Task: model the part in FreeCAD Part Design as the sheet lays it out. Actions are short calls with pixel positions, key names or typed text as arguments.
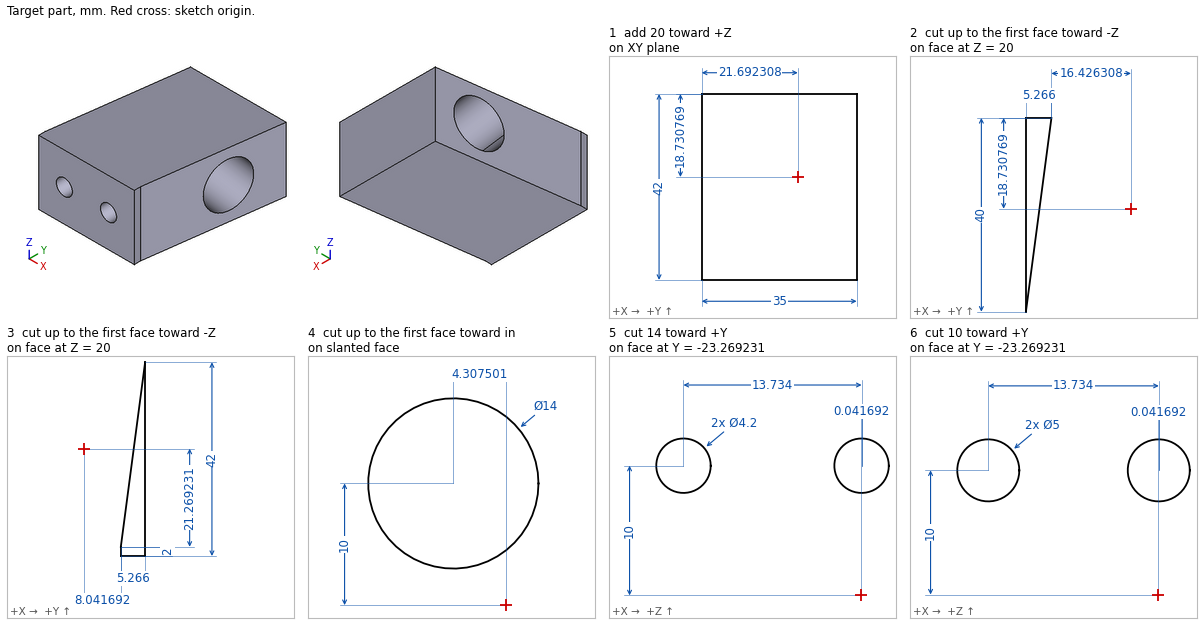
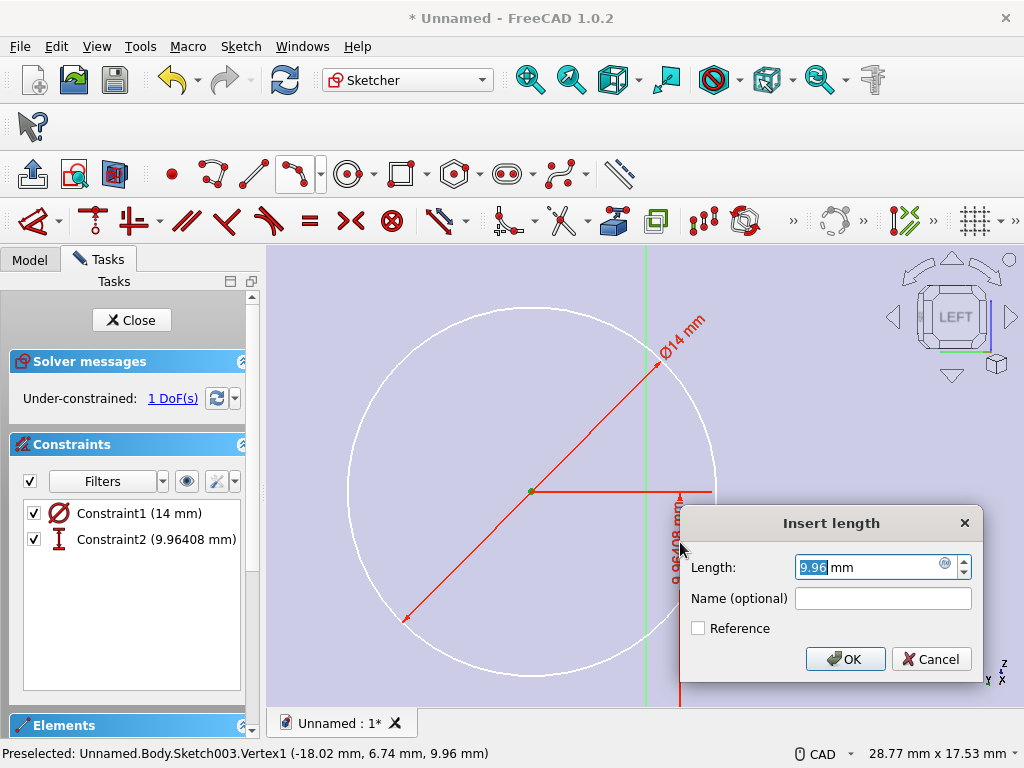
text(10)
key(Return)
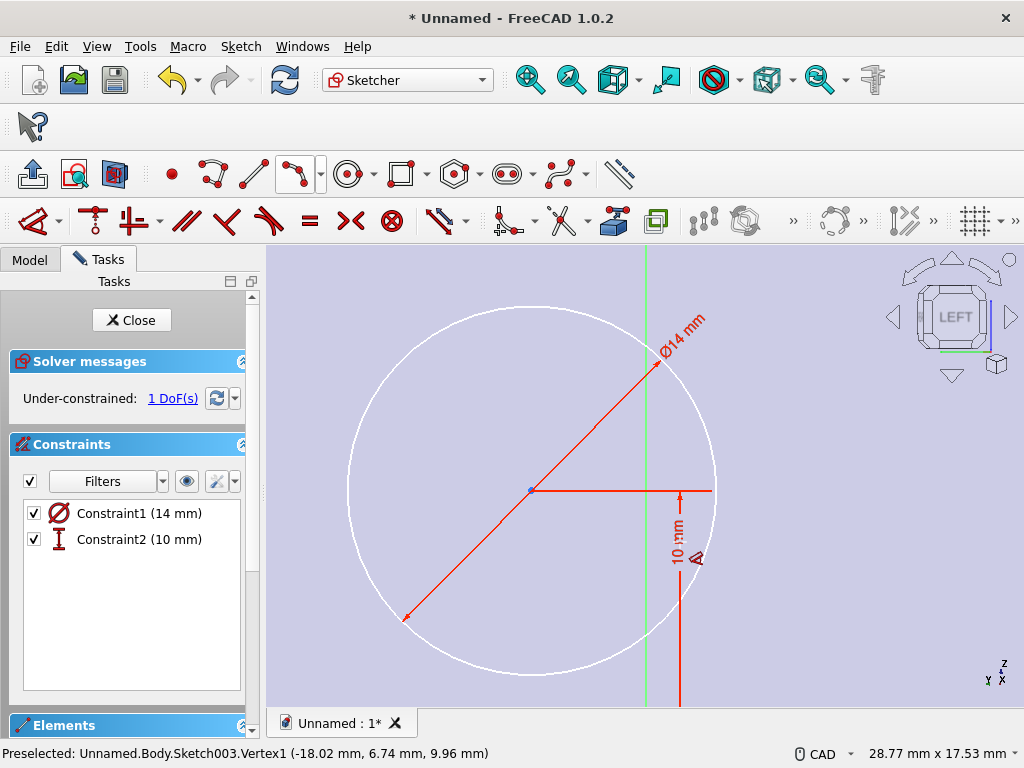
click(532, 491)
click(589, 457)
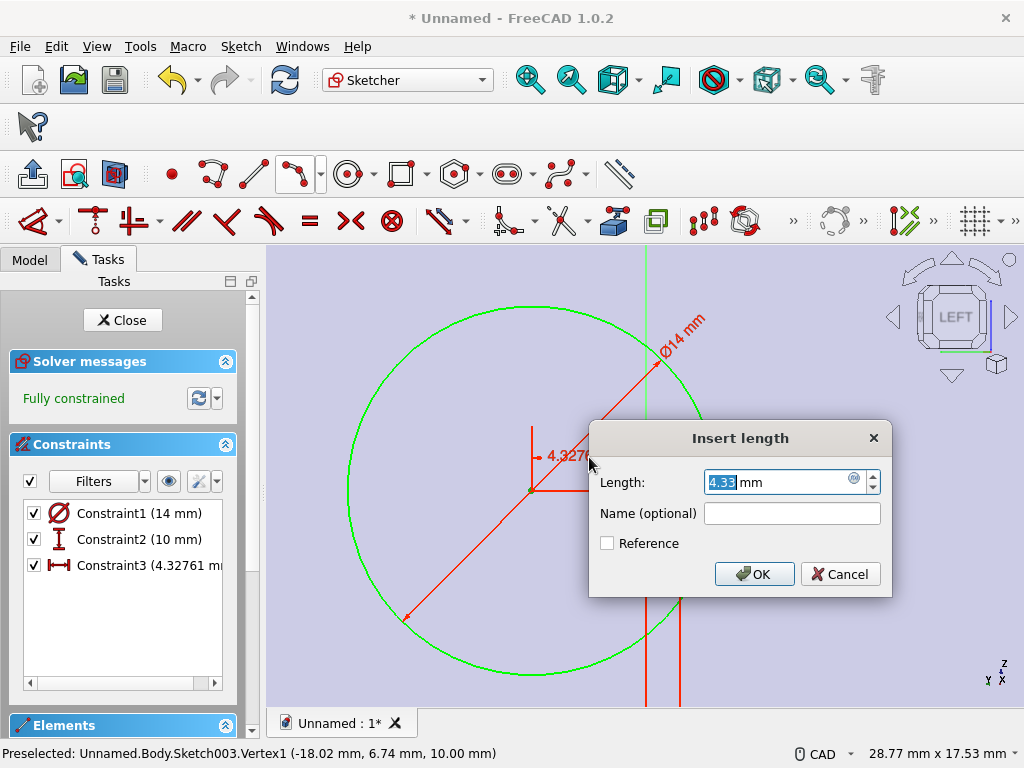
text(4.307501)
key(Return)
key(Escape)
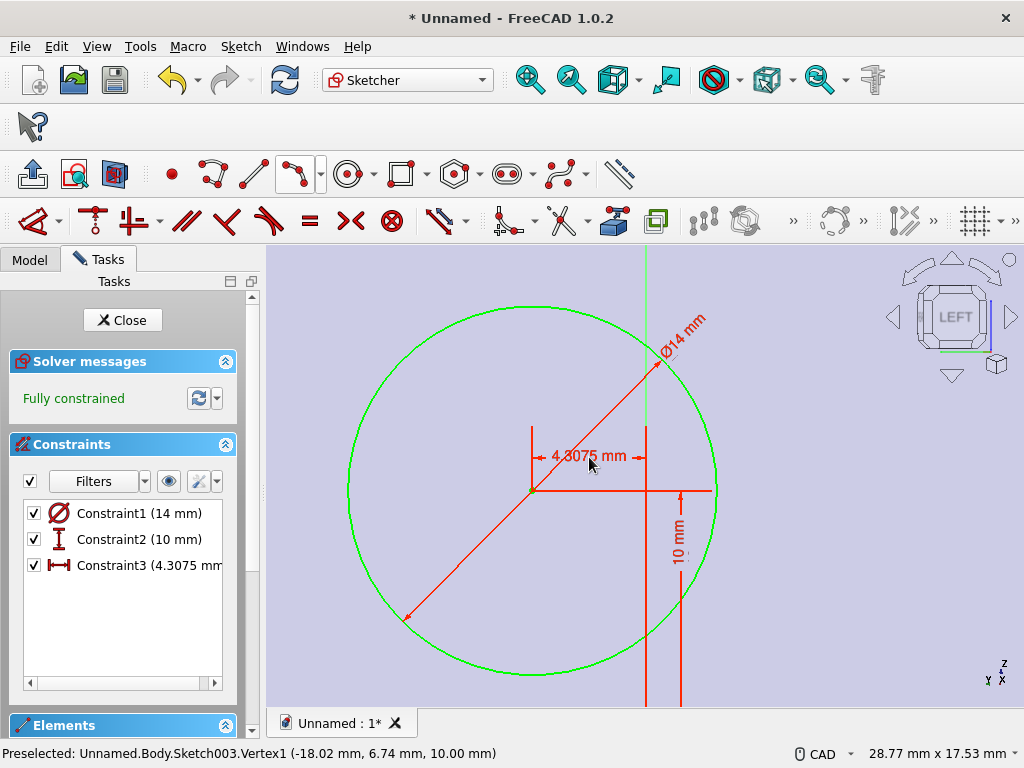
click(123, 320)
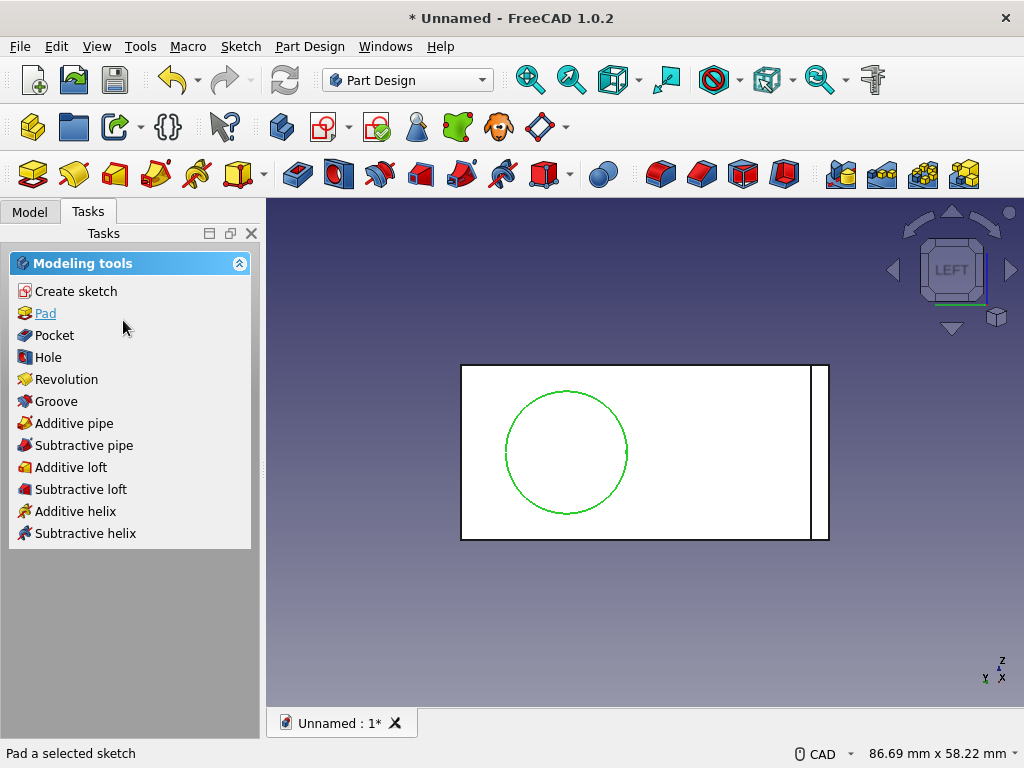
click(298, 174)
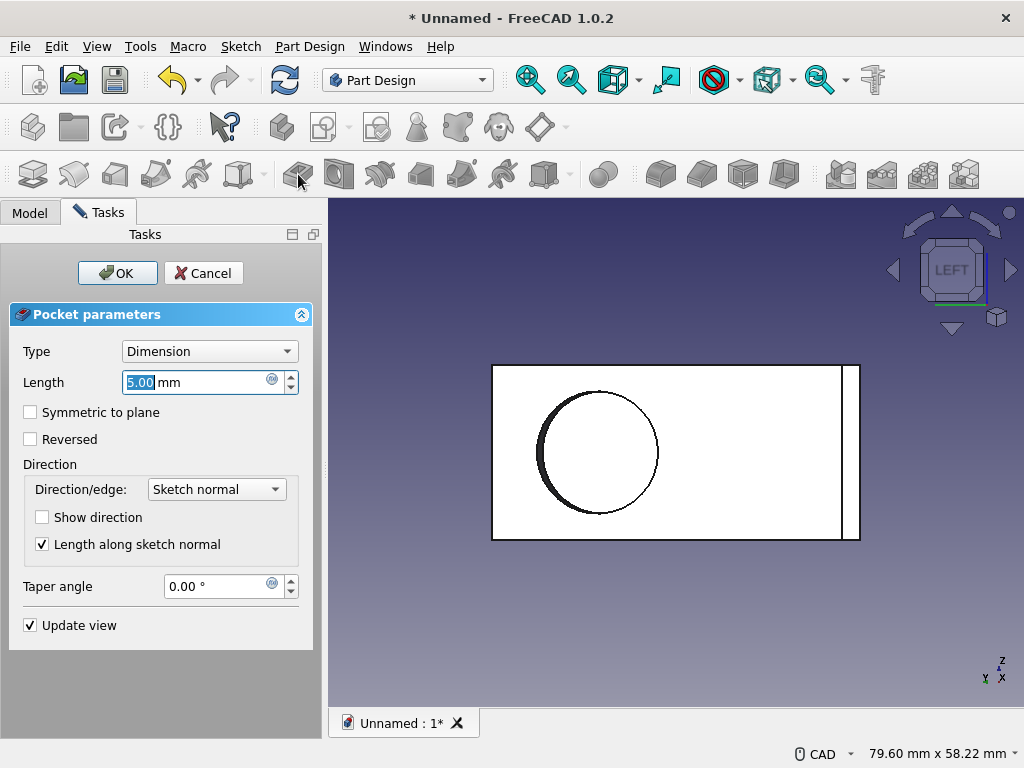
click(210, 352)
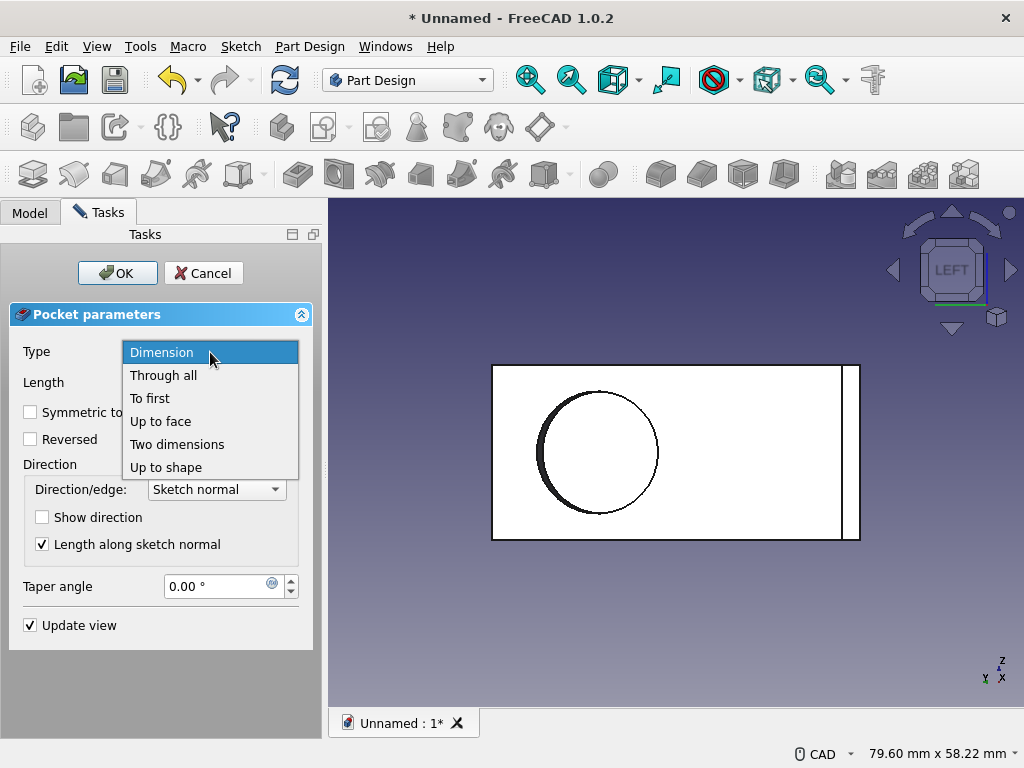
click(208, 398)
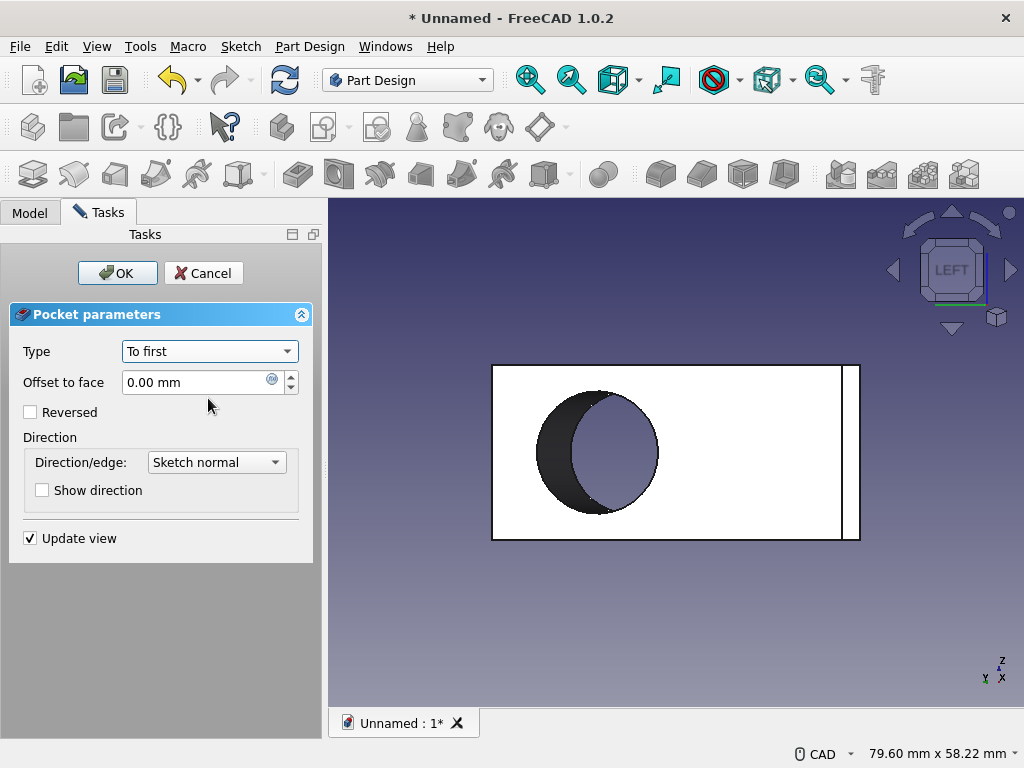
click(118, 273)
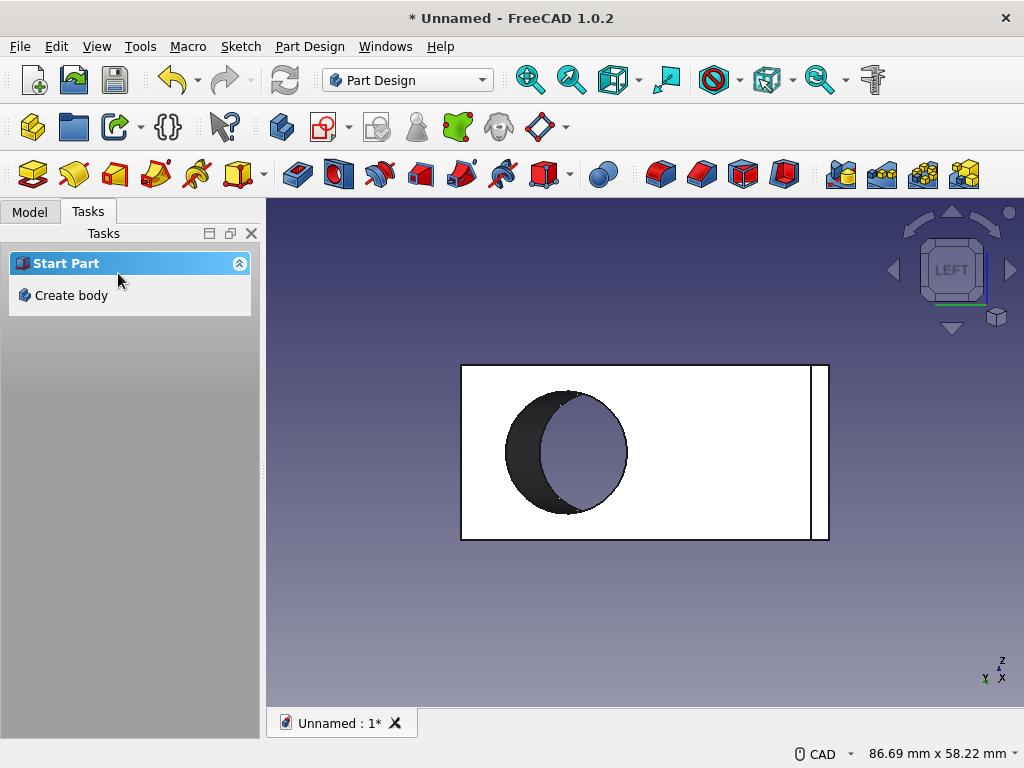
key(0)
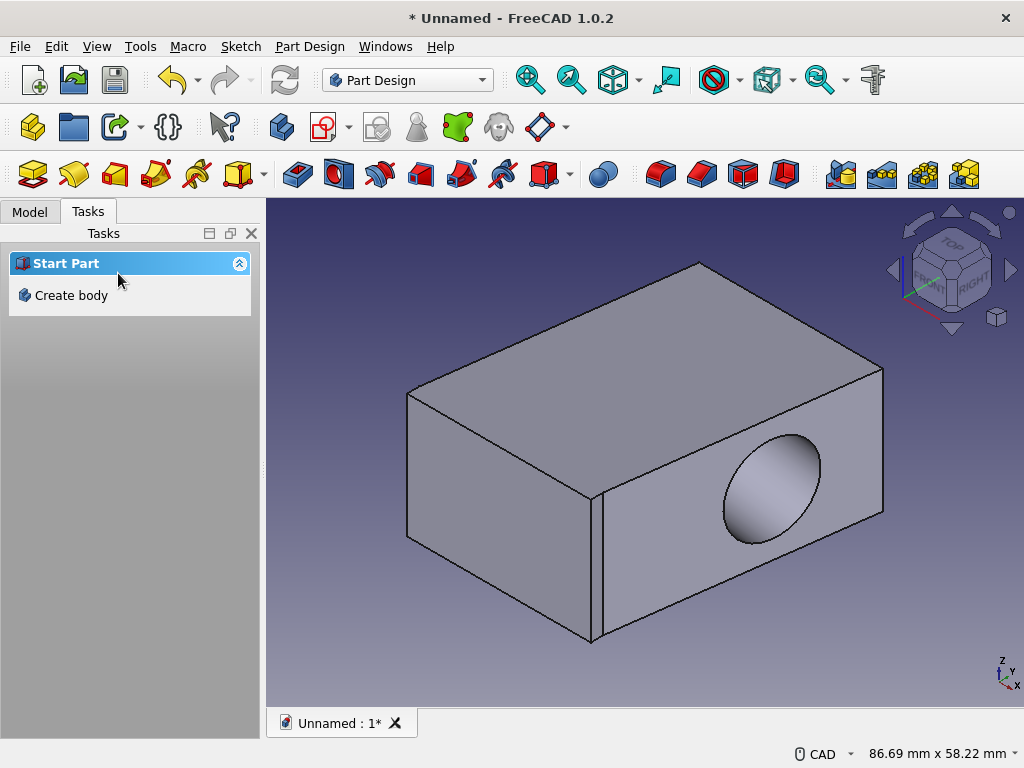
click(525, 532)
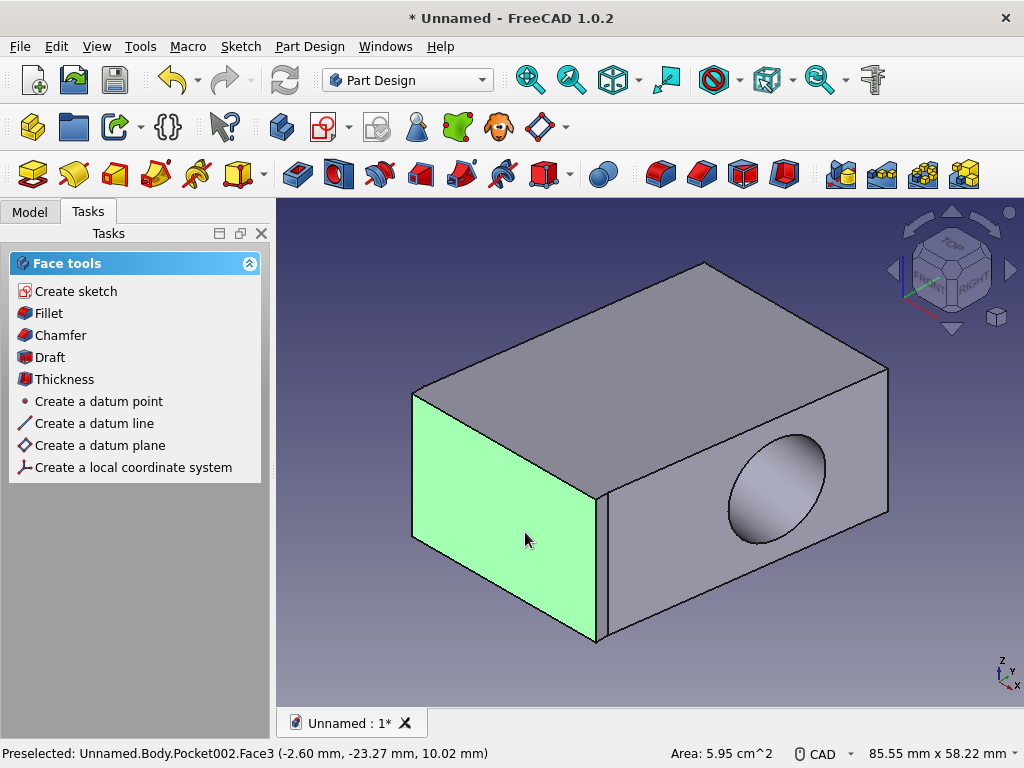
click(322, 128)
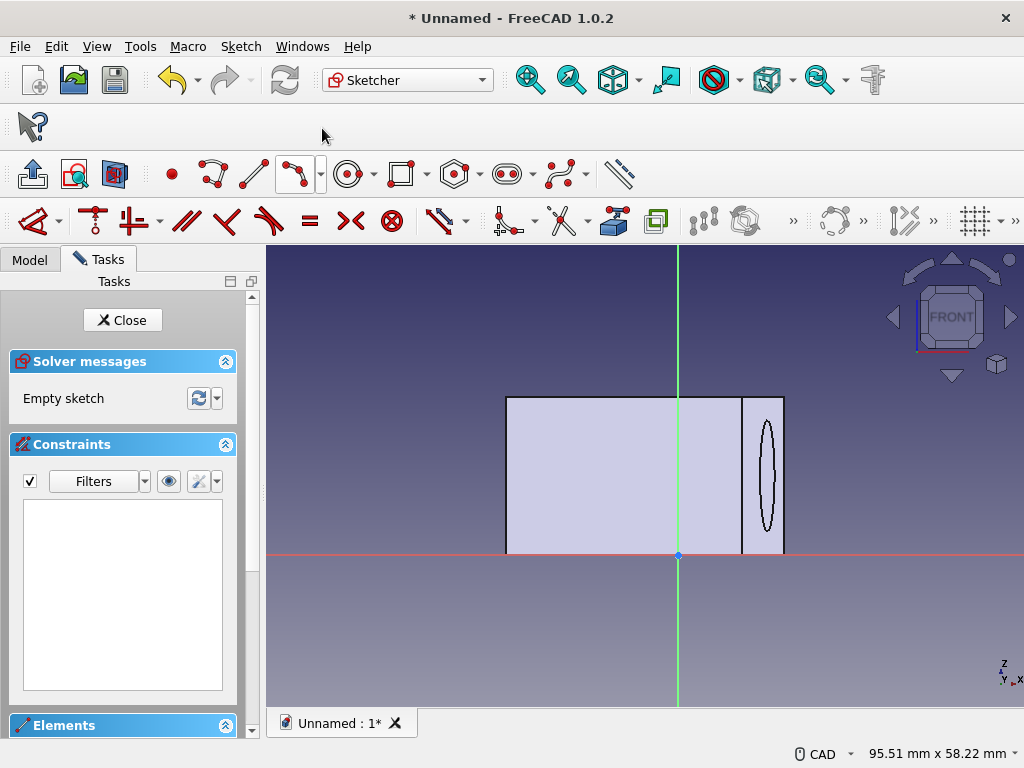
scroll(652, 526, up, 5)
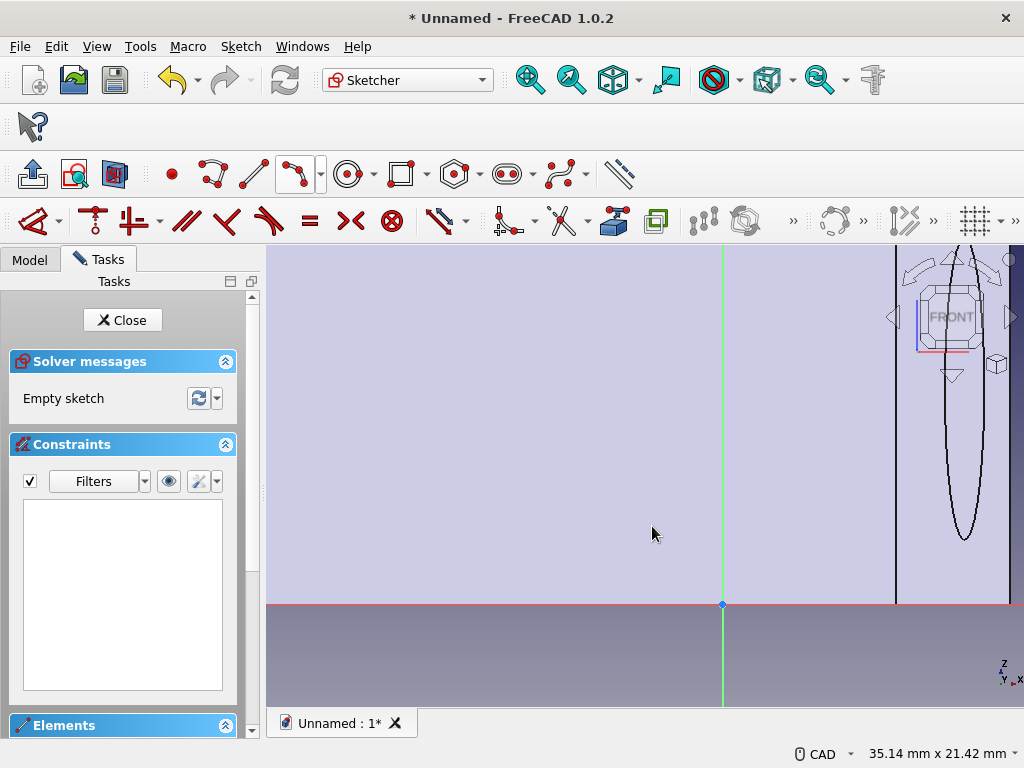
click(348, 174)